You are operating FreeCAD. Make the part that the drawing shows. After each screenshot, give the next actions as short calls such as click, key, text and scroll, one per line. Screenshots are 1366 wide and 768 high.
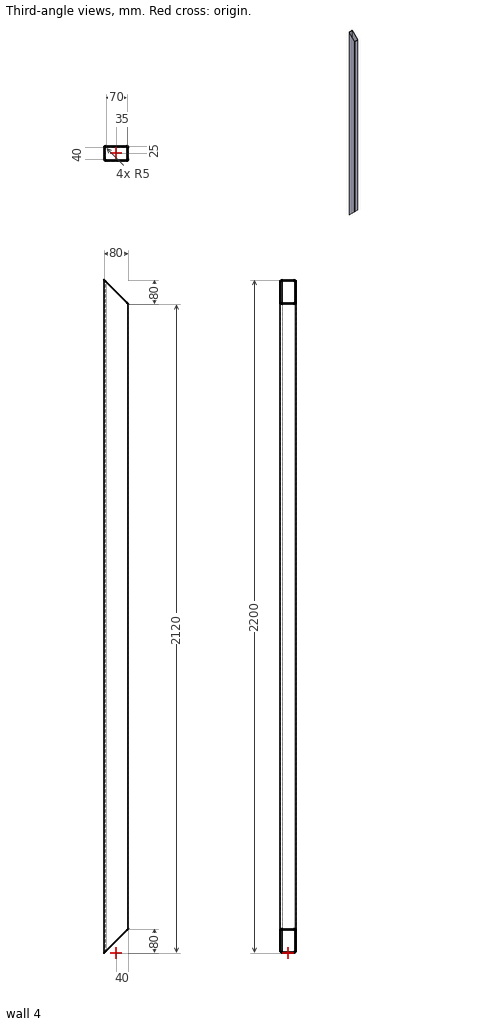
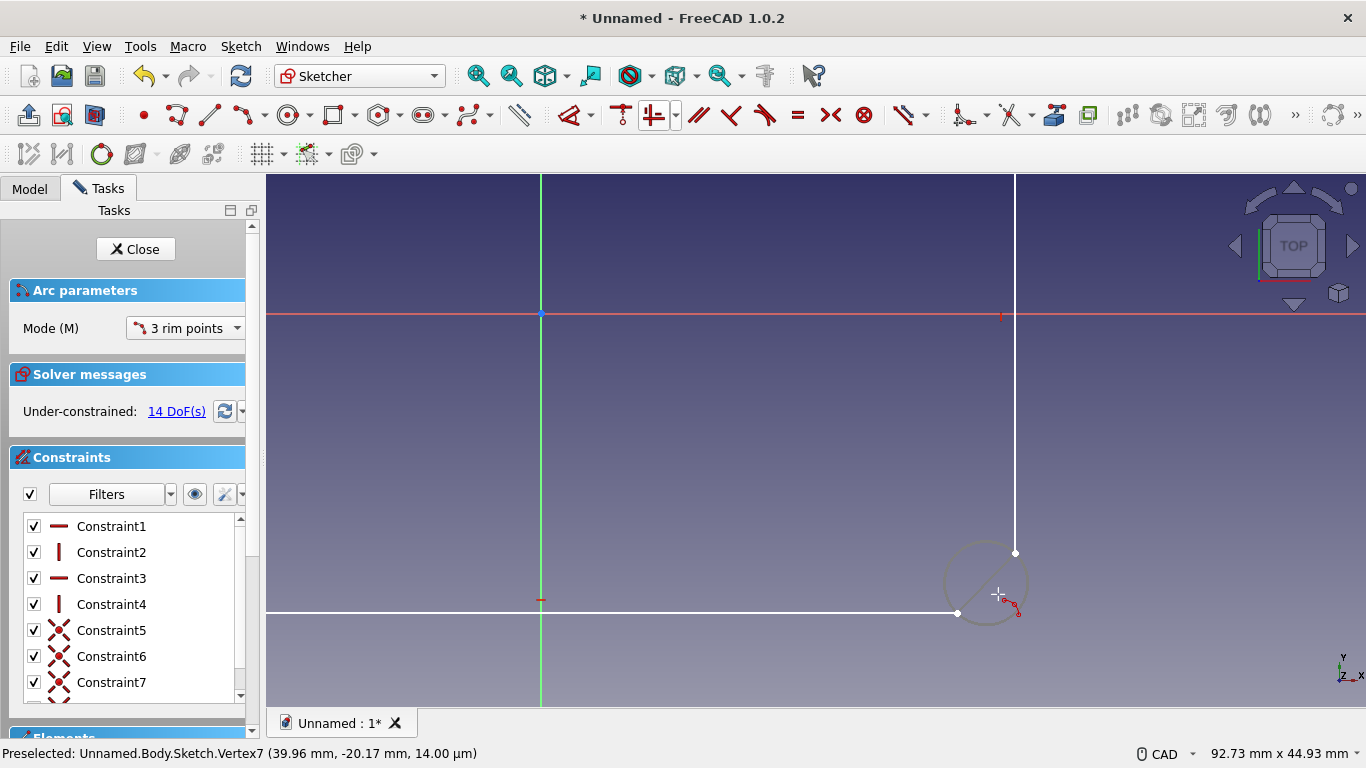
click(998, 593)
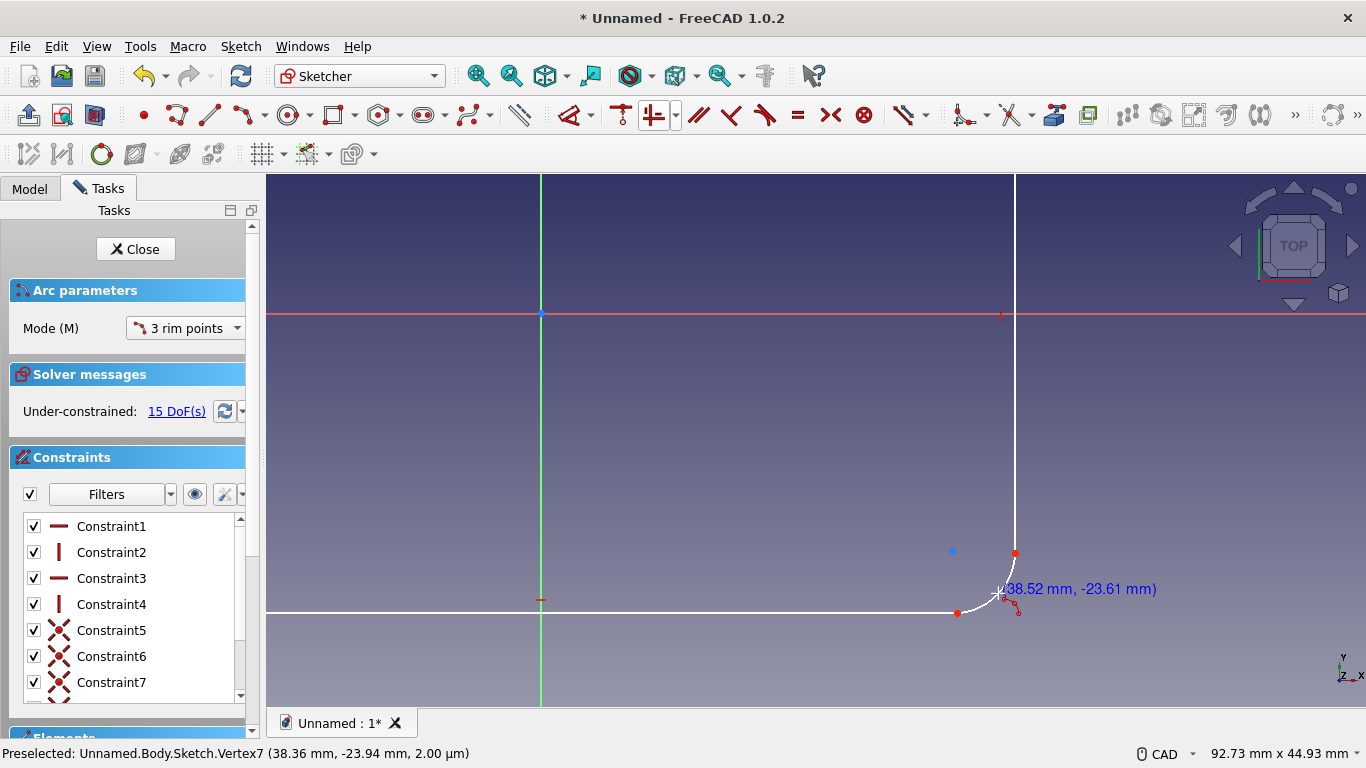
scroll(999, 594, down, 3)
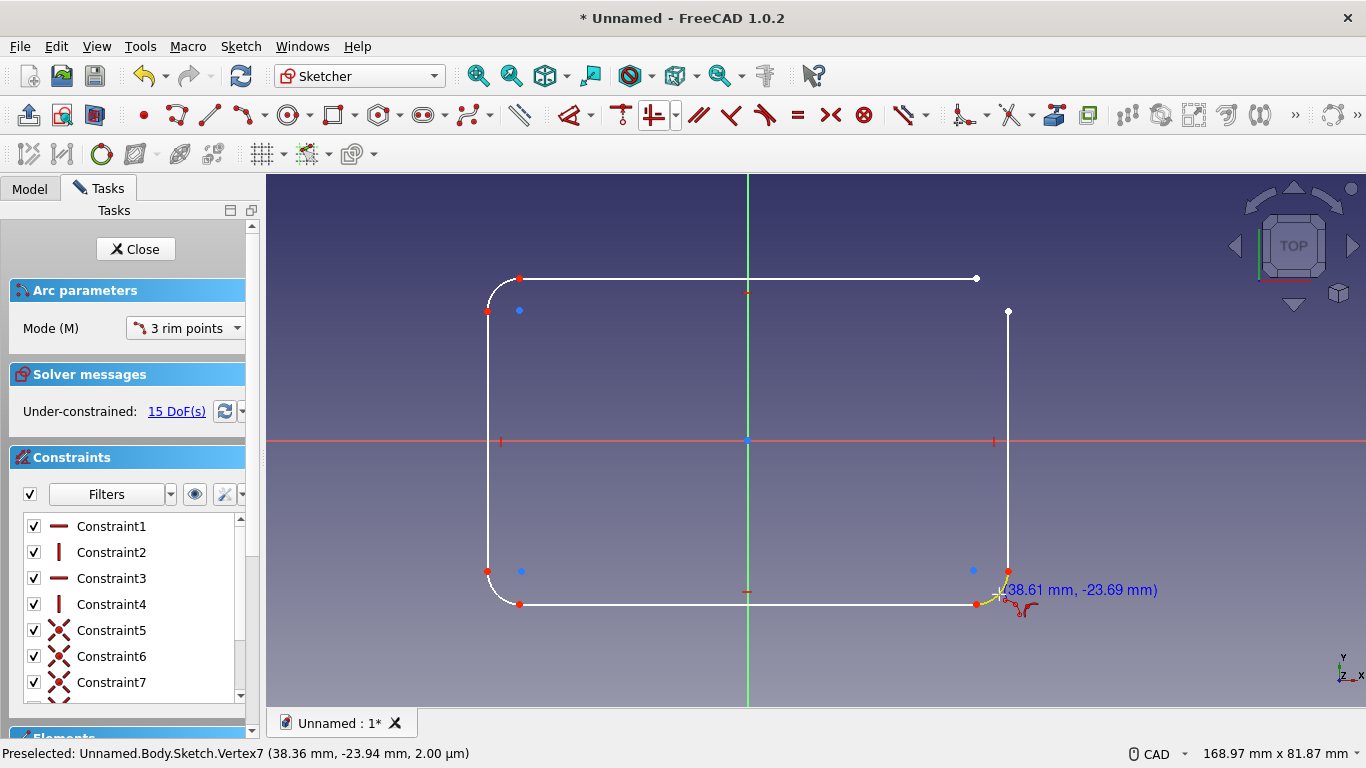
click(1008, 312)
click(976, 279)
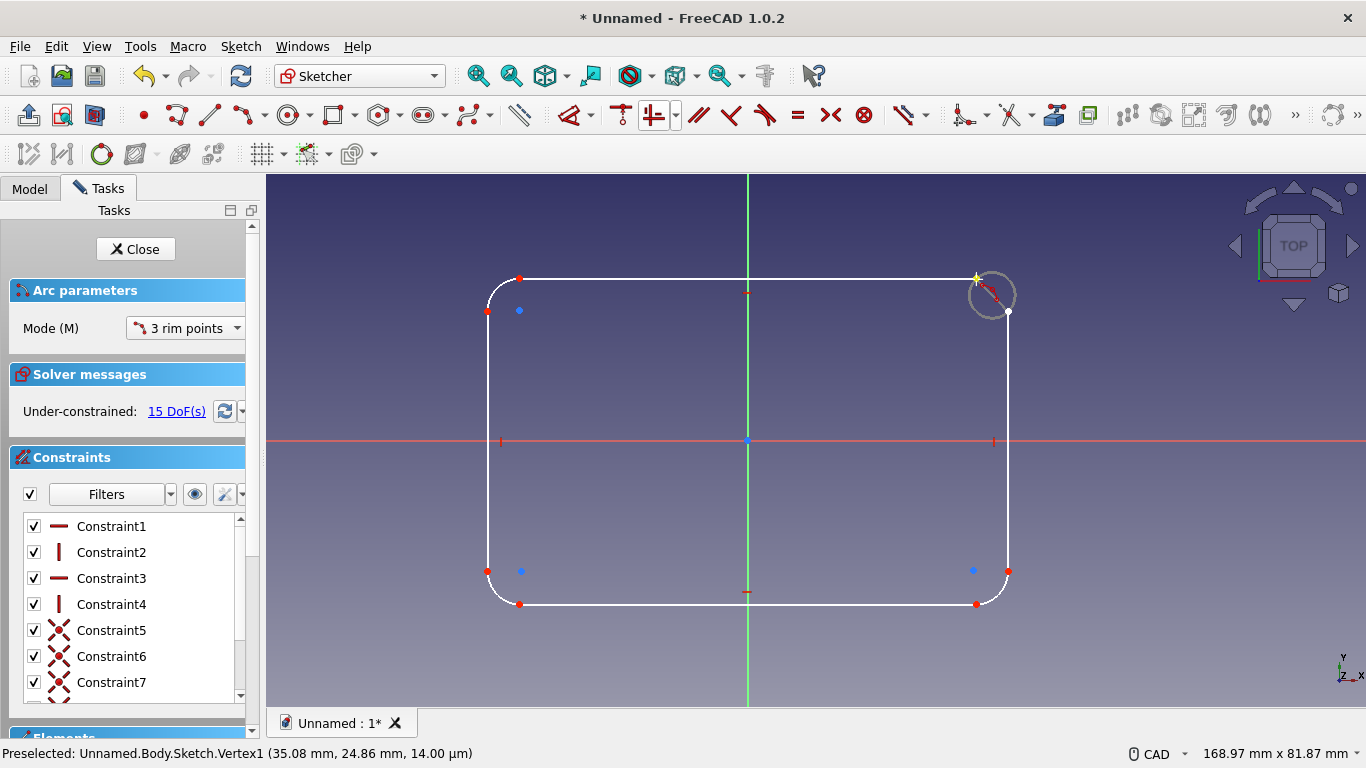
scroll(999, 287, up, 3)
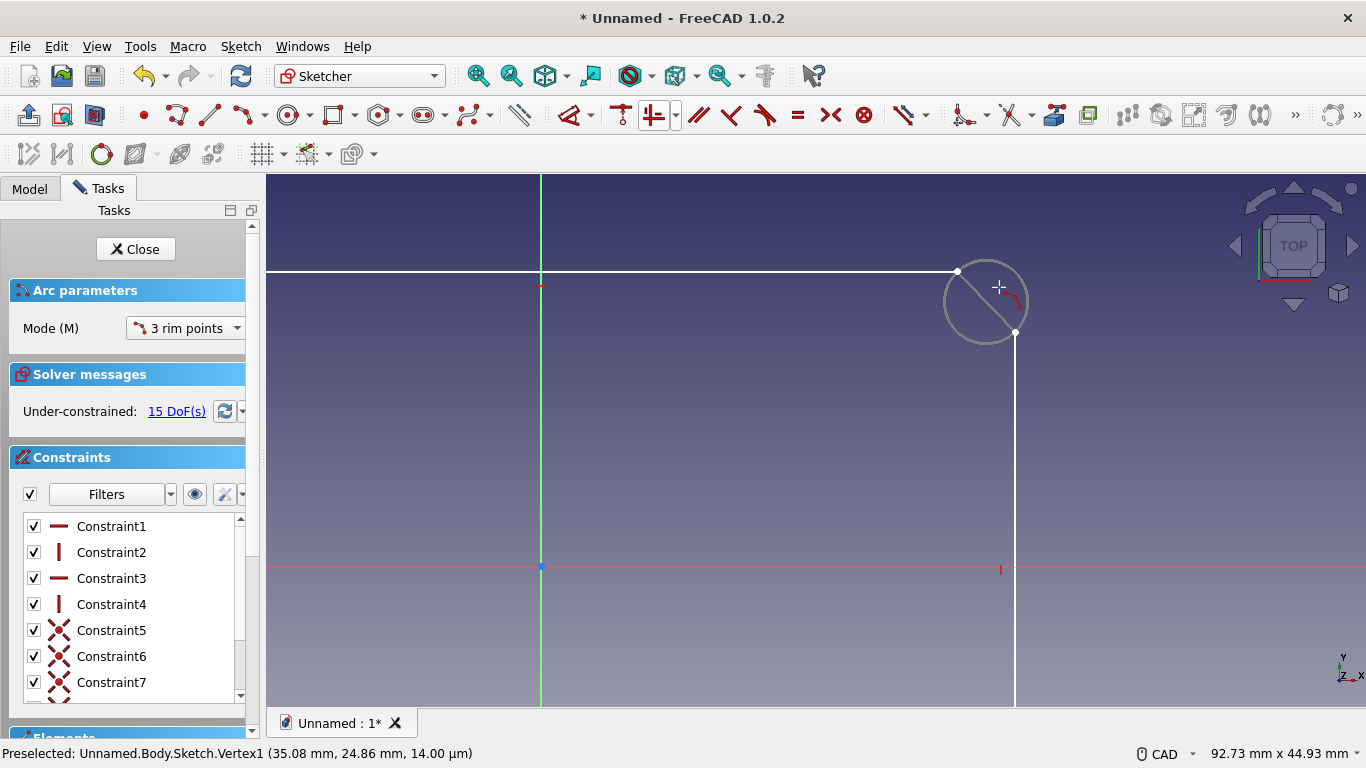
click(998, 288)
key(Escape)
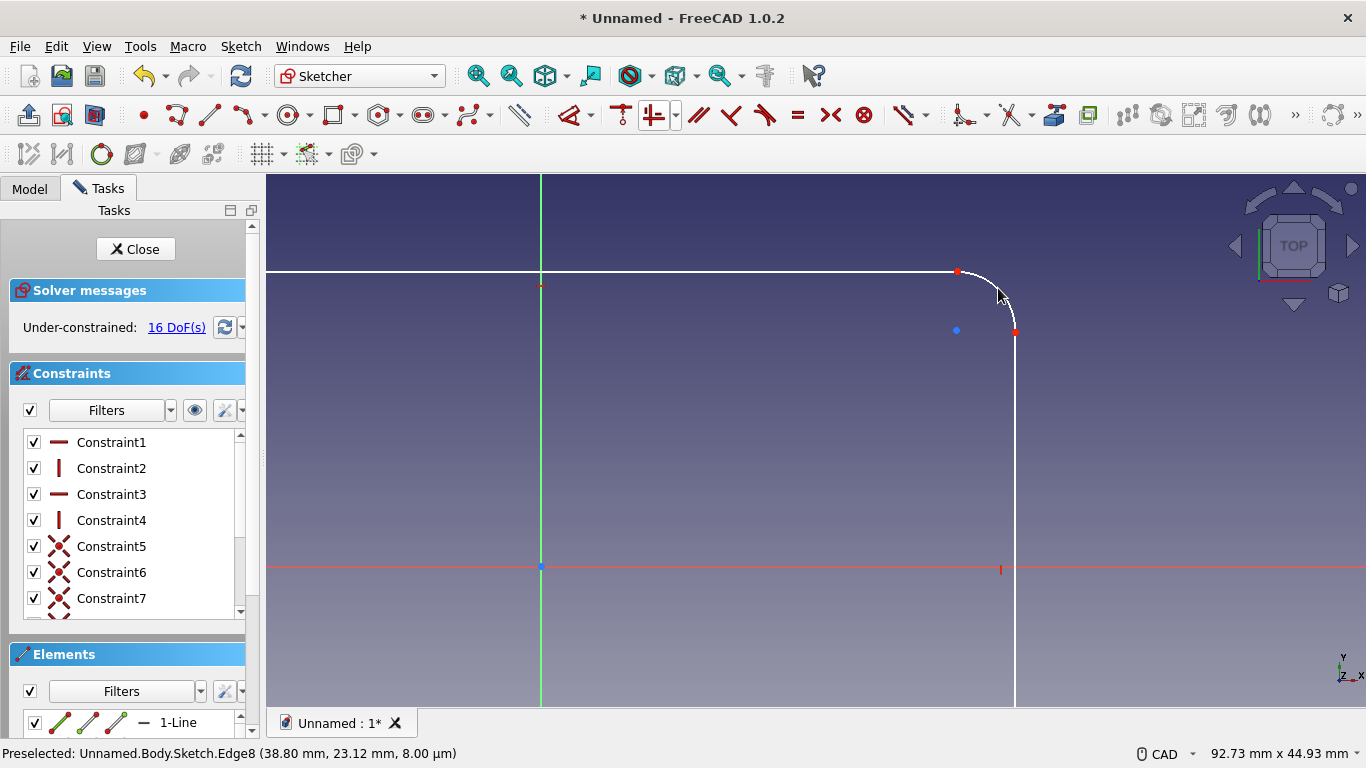
click(708, 272)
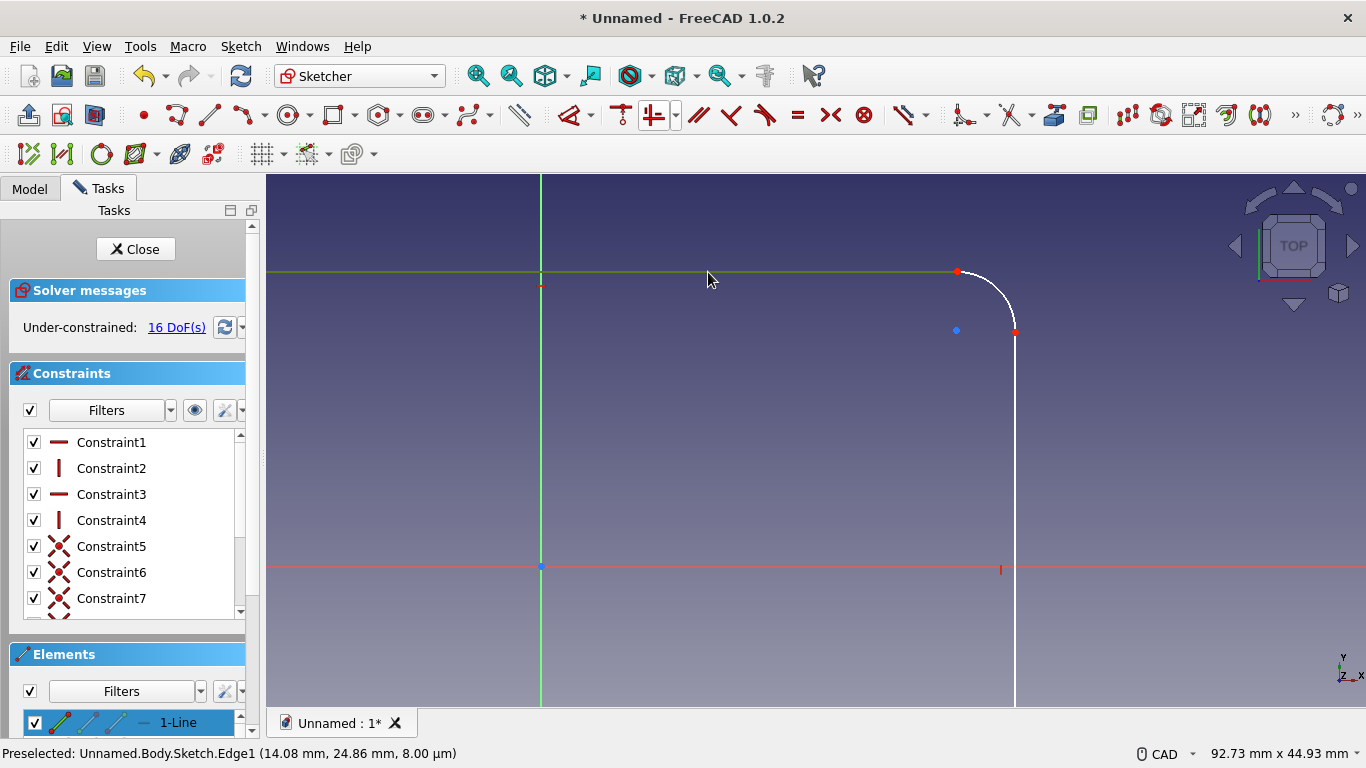
scroll(999, 287, down, 3)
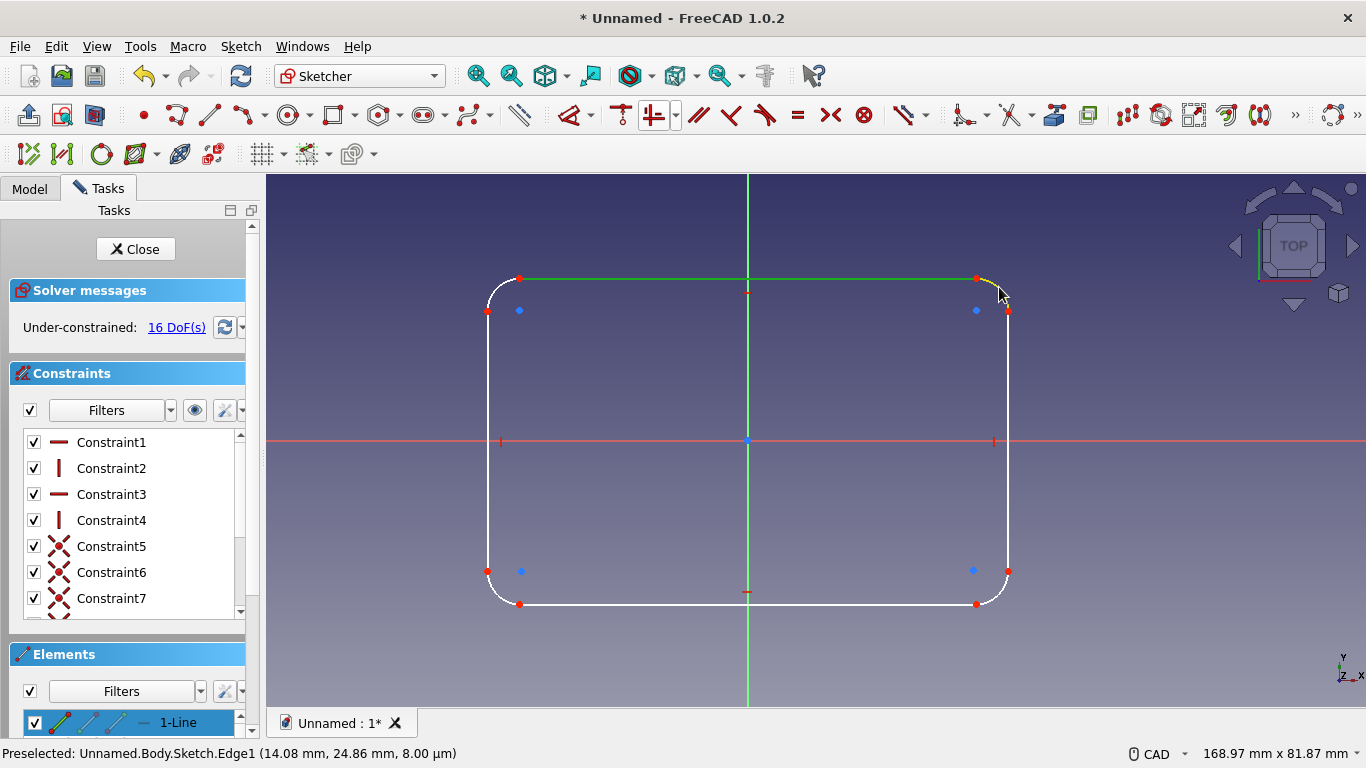
click(505, 283)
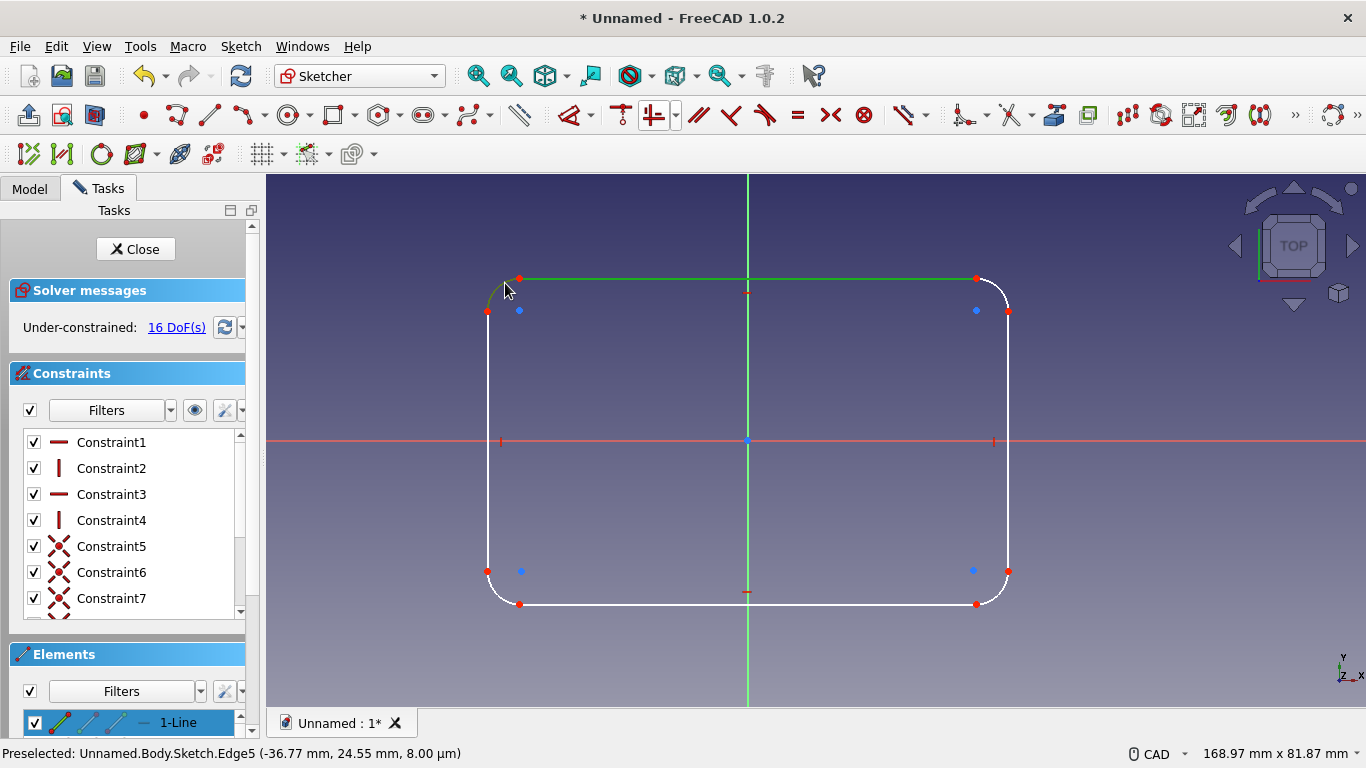
click(765, 116)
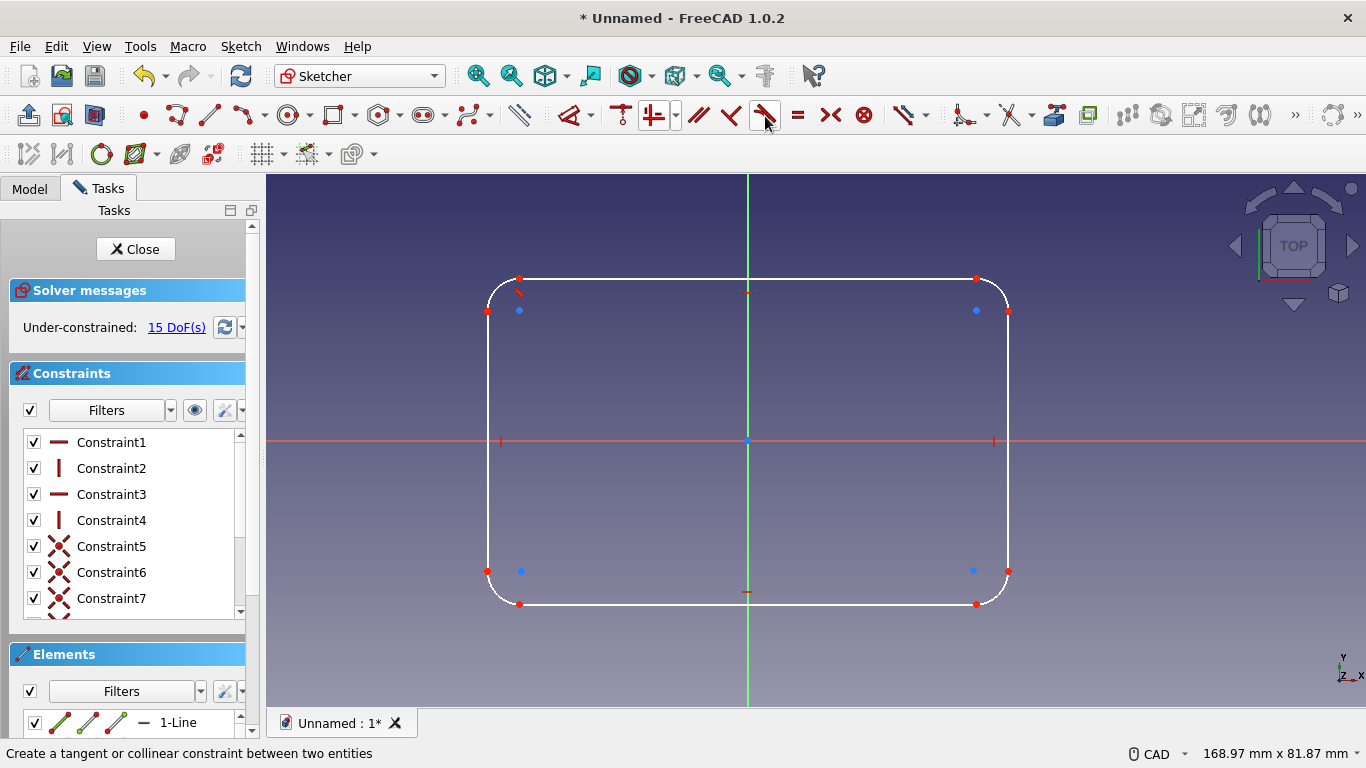
click(839, 279)